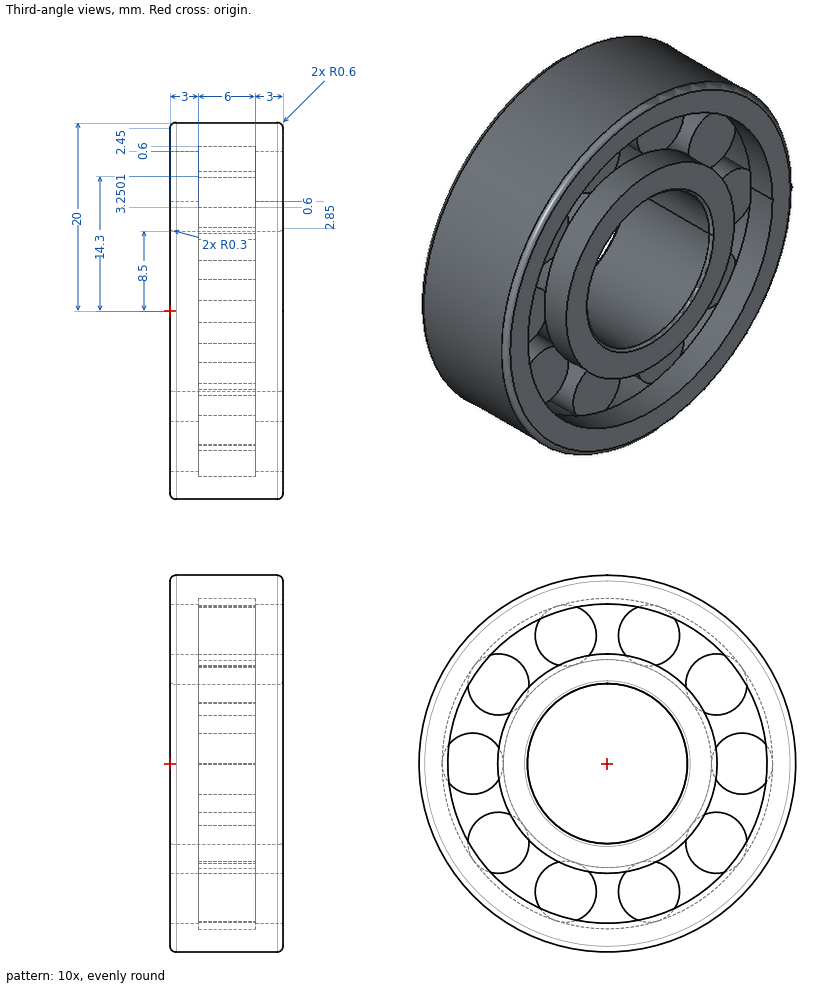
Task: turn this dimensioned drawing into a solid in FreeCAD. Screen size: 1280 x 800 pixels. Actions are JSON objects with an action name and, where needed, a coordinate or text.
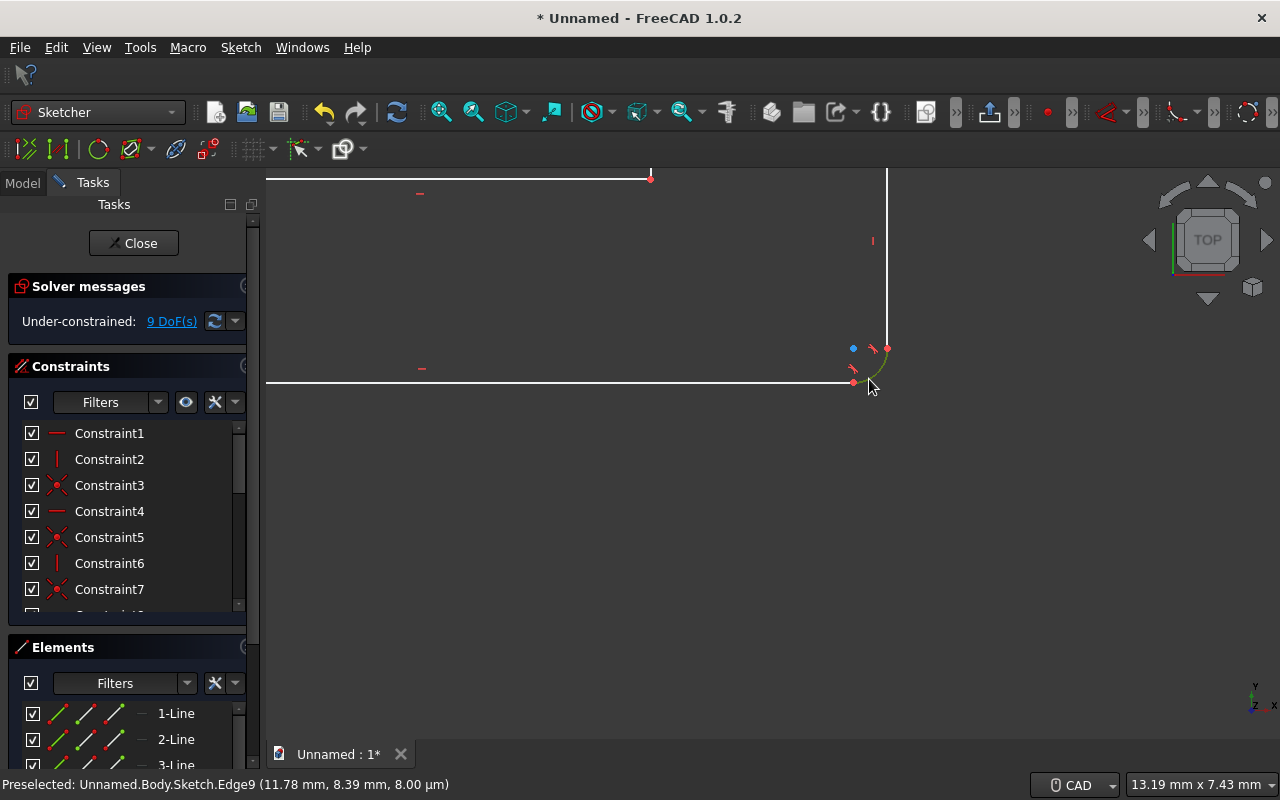
{"action": "scroll", "coordinate": [870, 381], "scroll_direction": "down", "scroll_amount": 5}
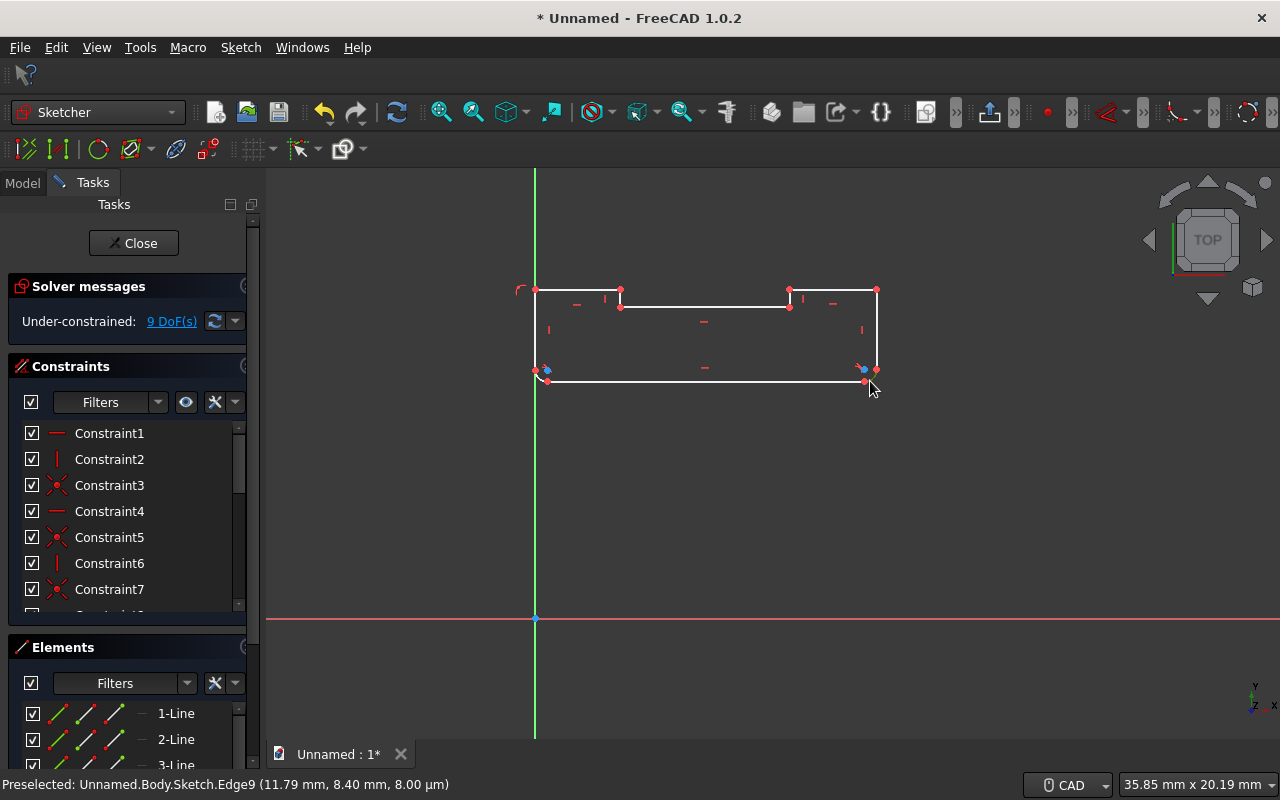
{"action": "scroll", "coordinate": [537, 375], "scroll_direction": "up", "scroll_amount": 5}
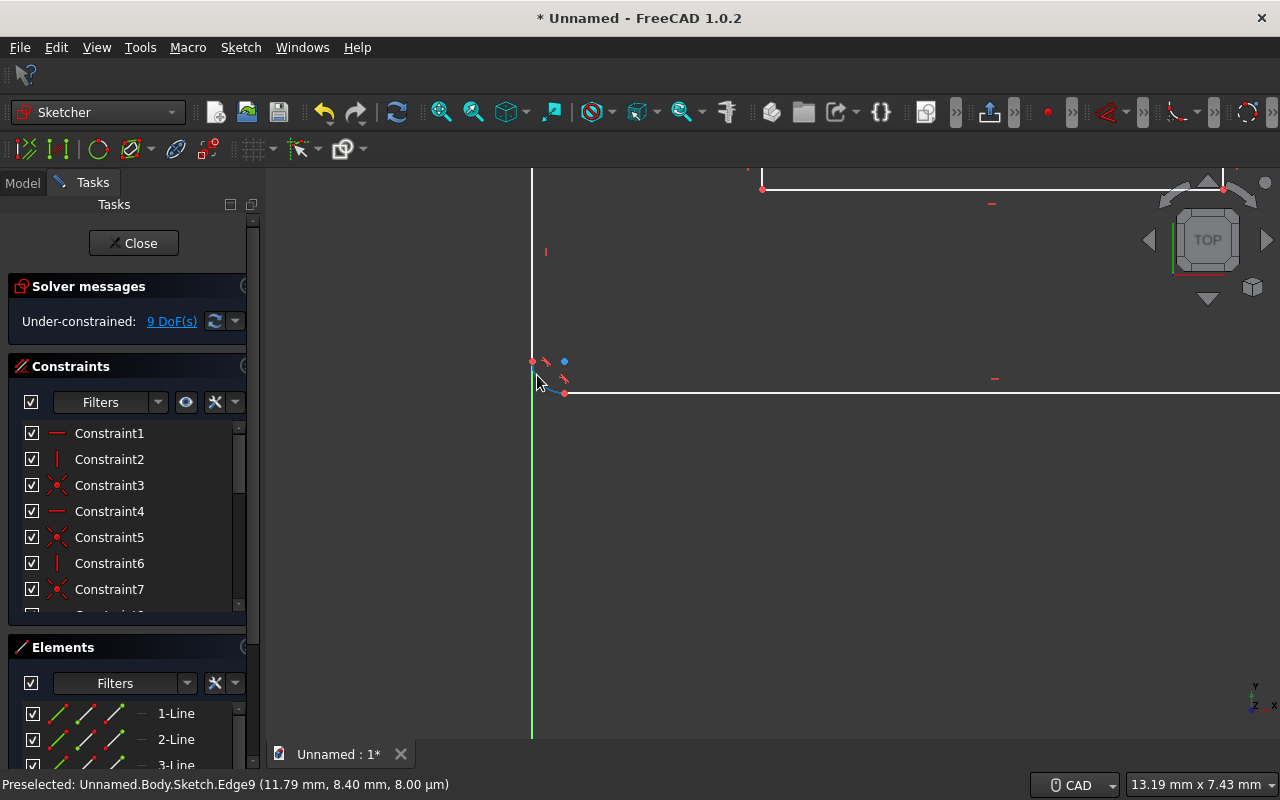
{"action": "left_click", "coordinate": [536, 376]}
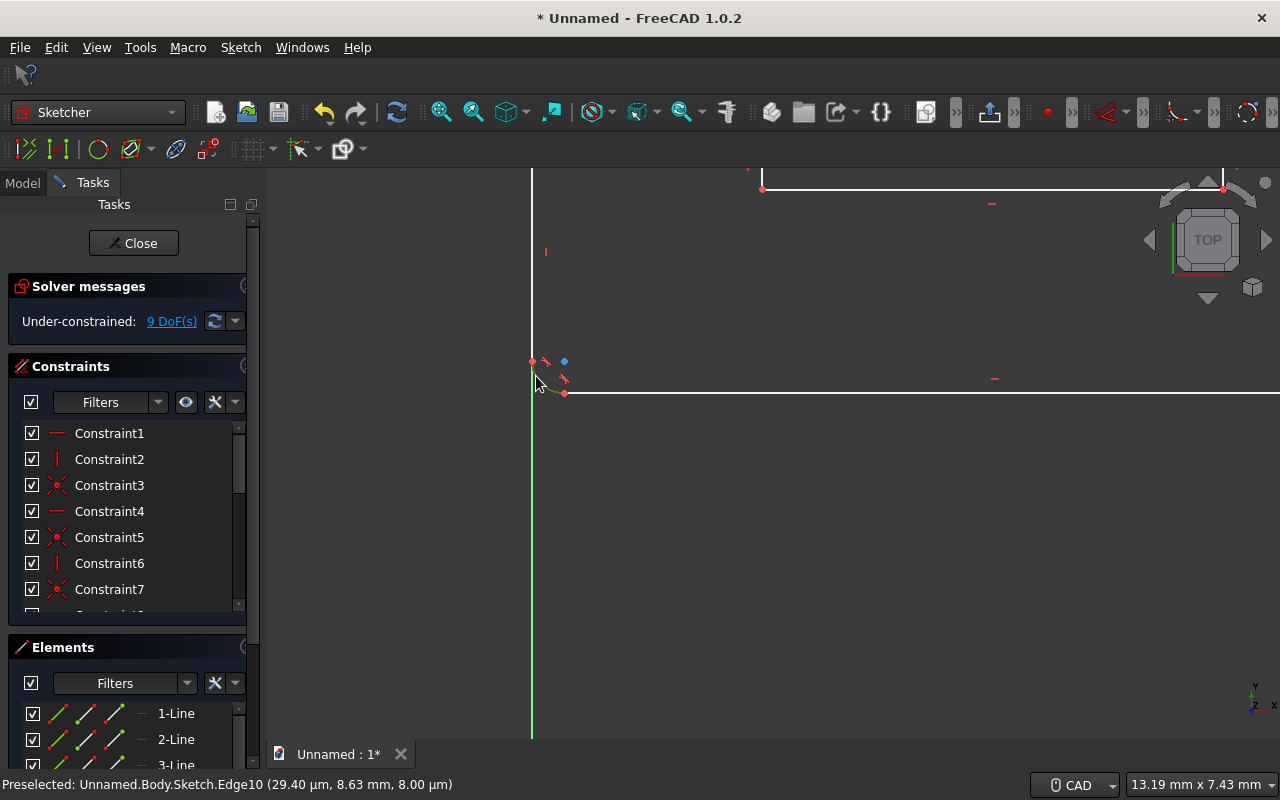
{"action": "key", "text": "e"}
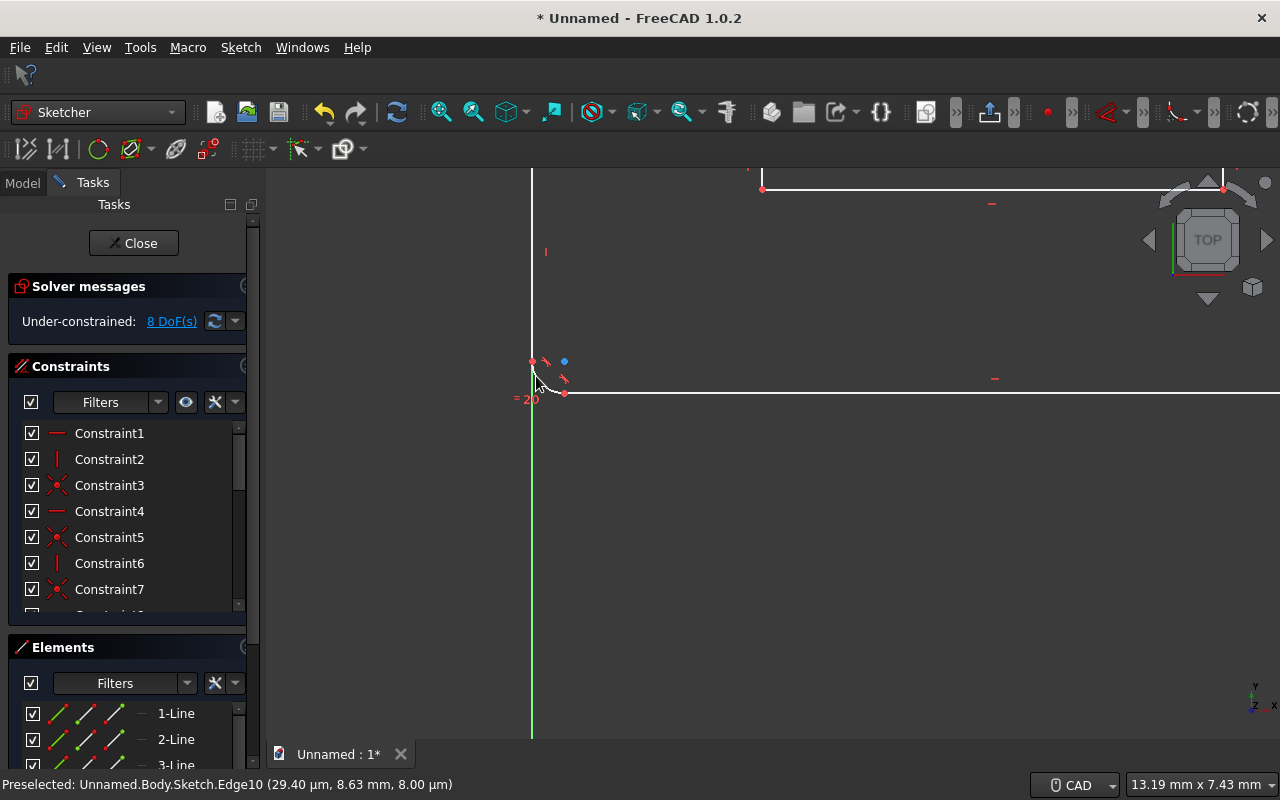
{"action": "scroll", "coordinate": [536, 375], "scroll_direction": "down", "scroll_amount": 5}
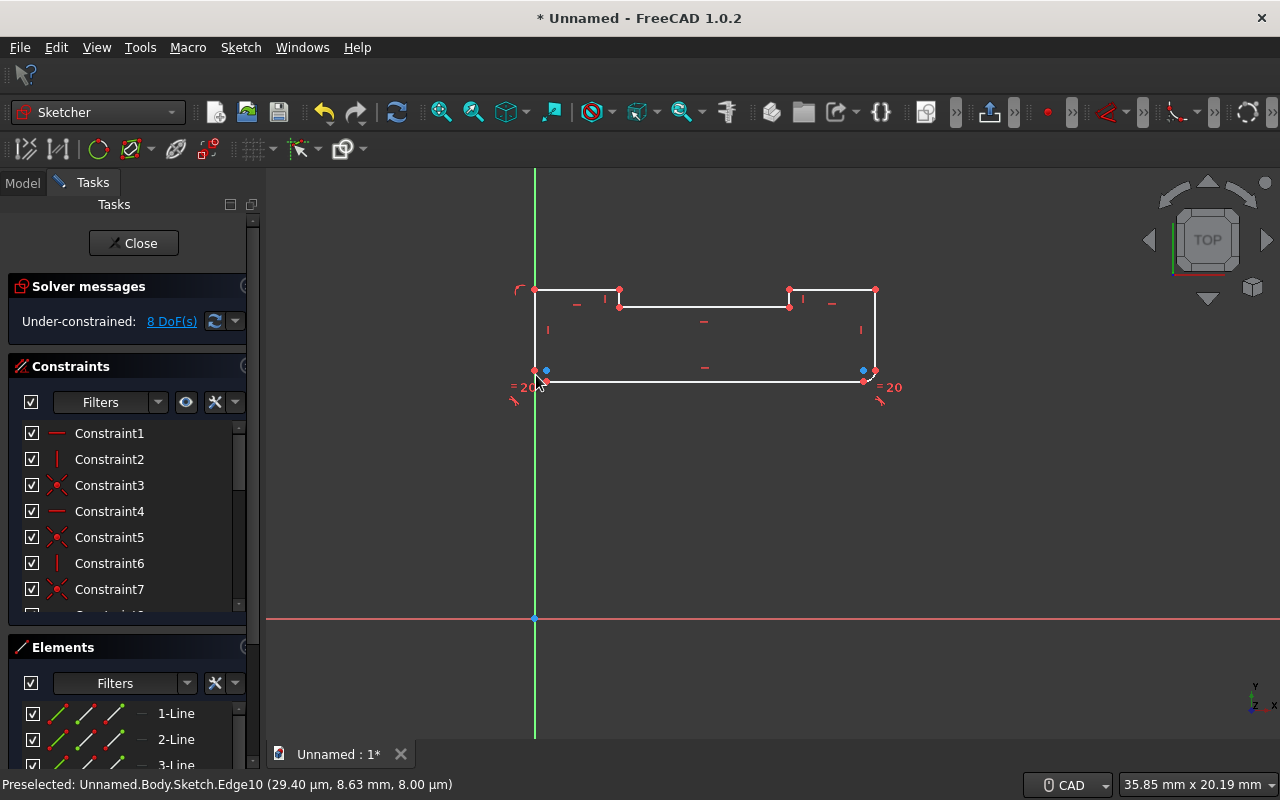
{"action": "scroll", "coordinate": [869, 381], "scroll_direction": "up", "scroll_amount": 8}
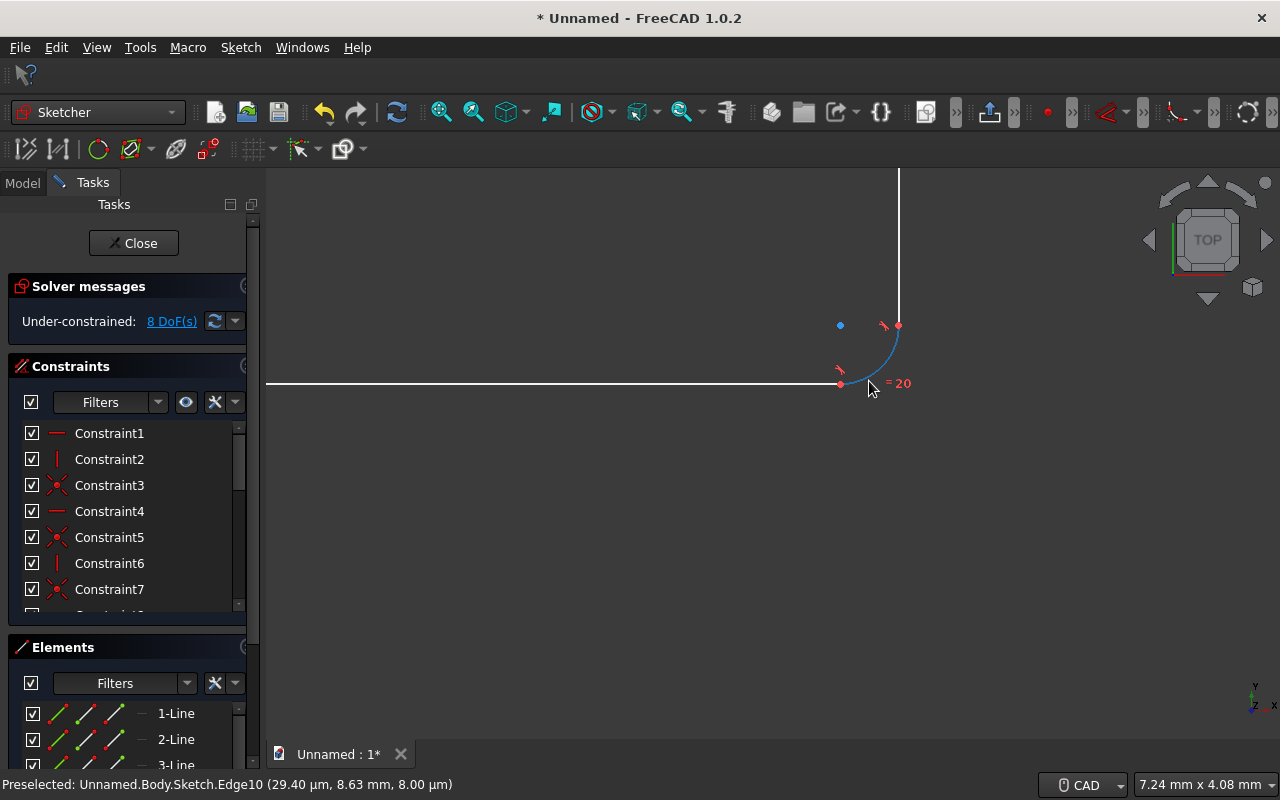
{"action": "left_click", "coordinate": [867, 378]}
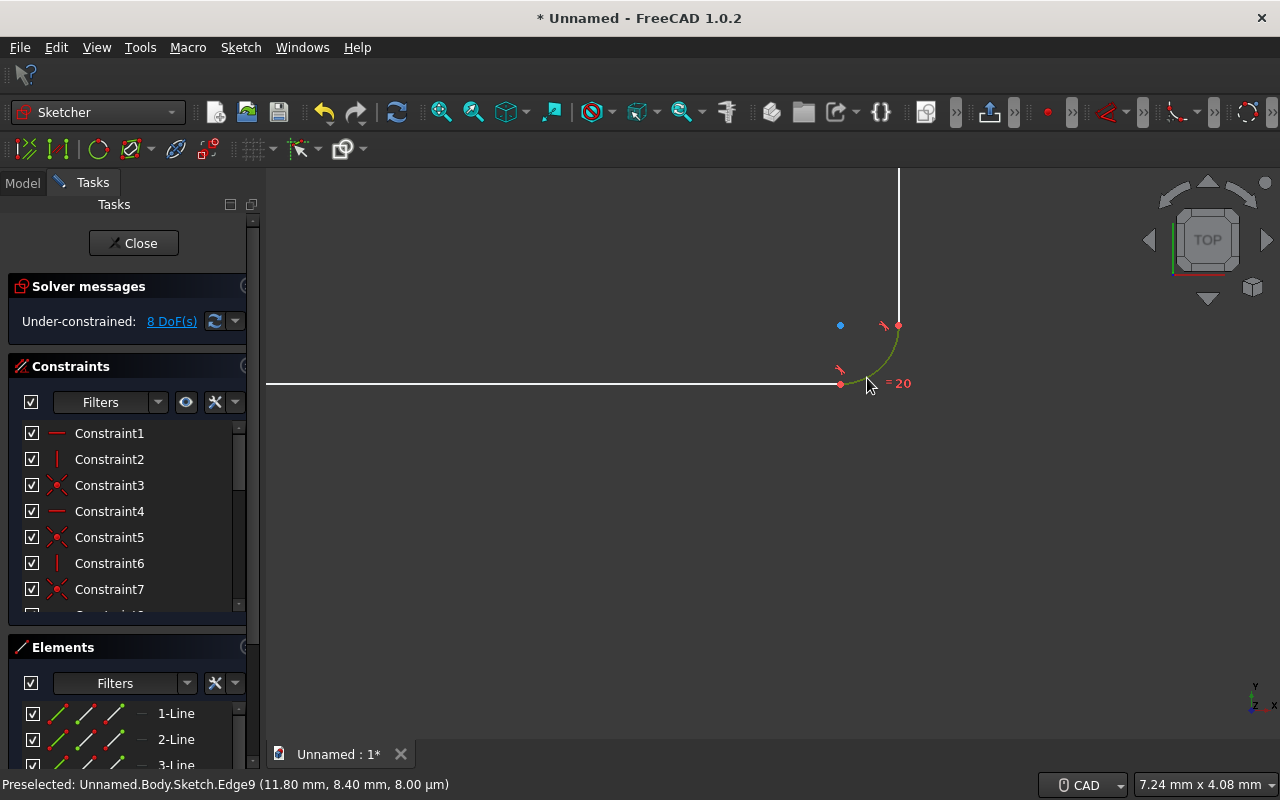
{"action": "key", "text": "k r"}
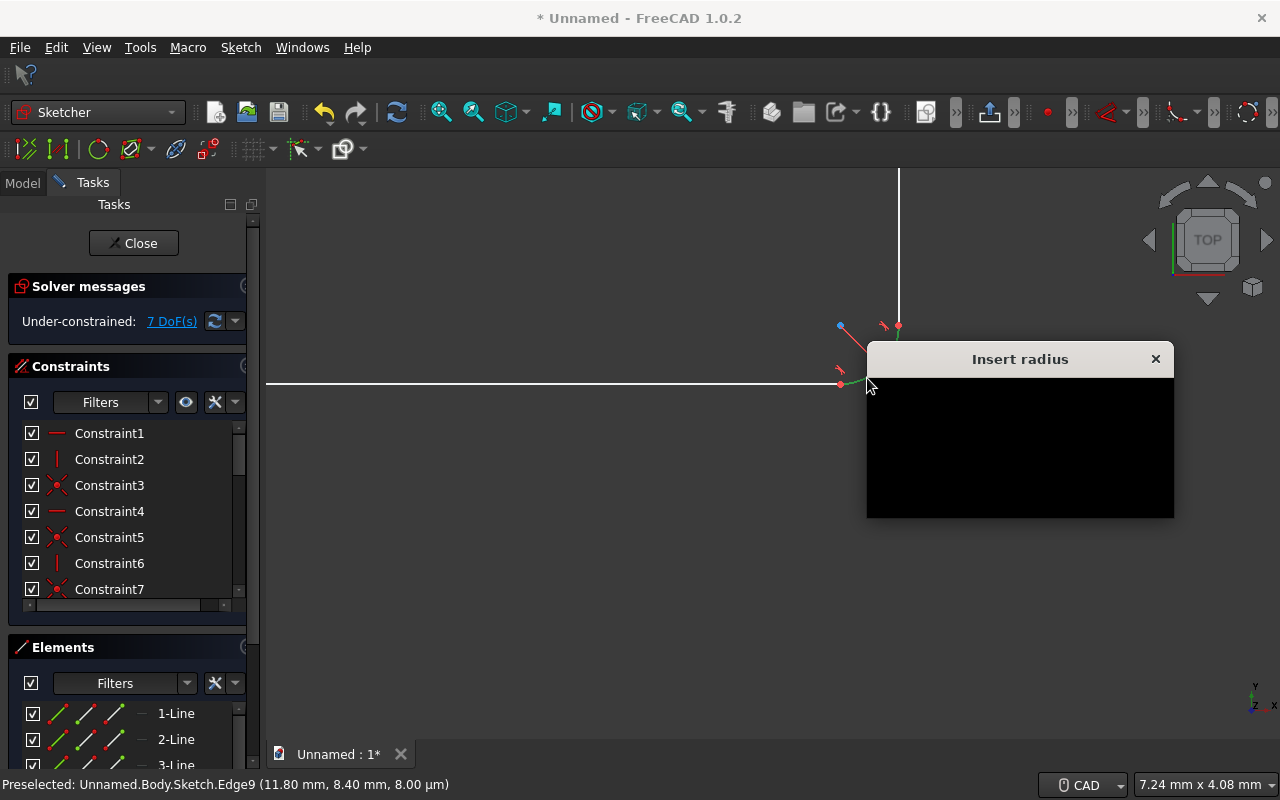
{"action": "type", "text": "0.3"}
{"action": "key", "text": "Return"}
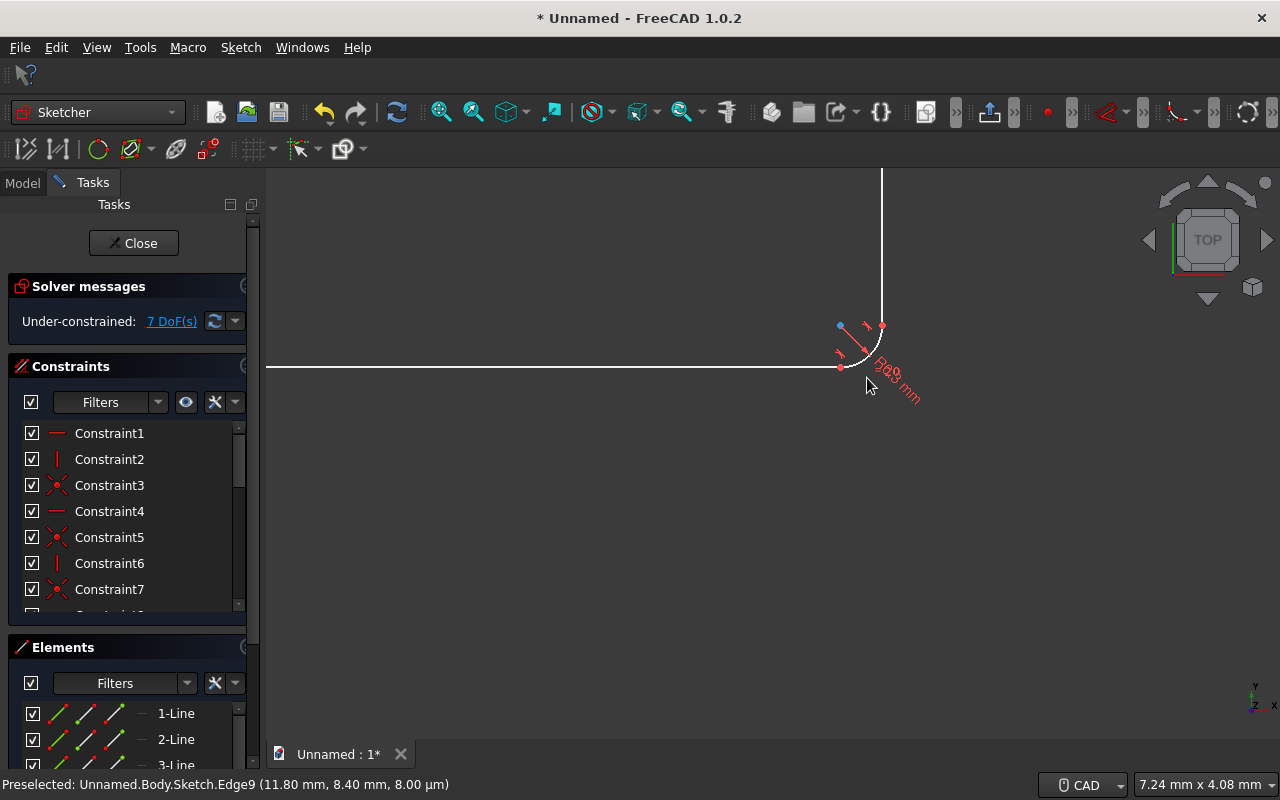
{"action": "scroll", "coordinate": [870, 381], "scroll_direction": "down", "scroll_amount": 8}